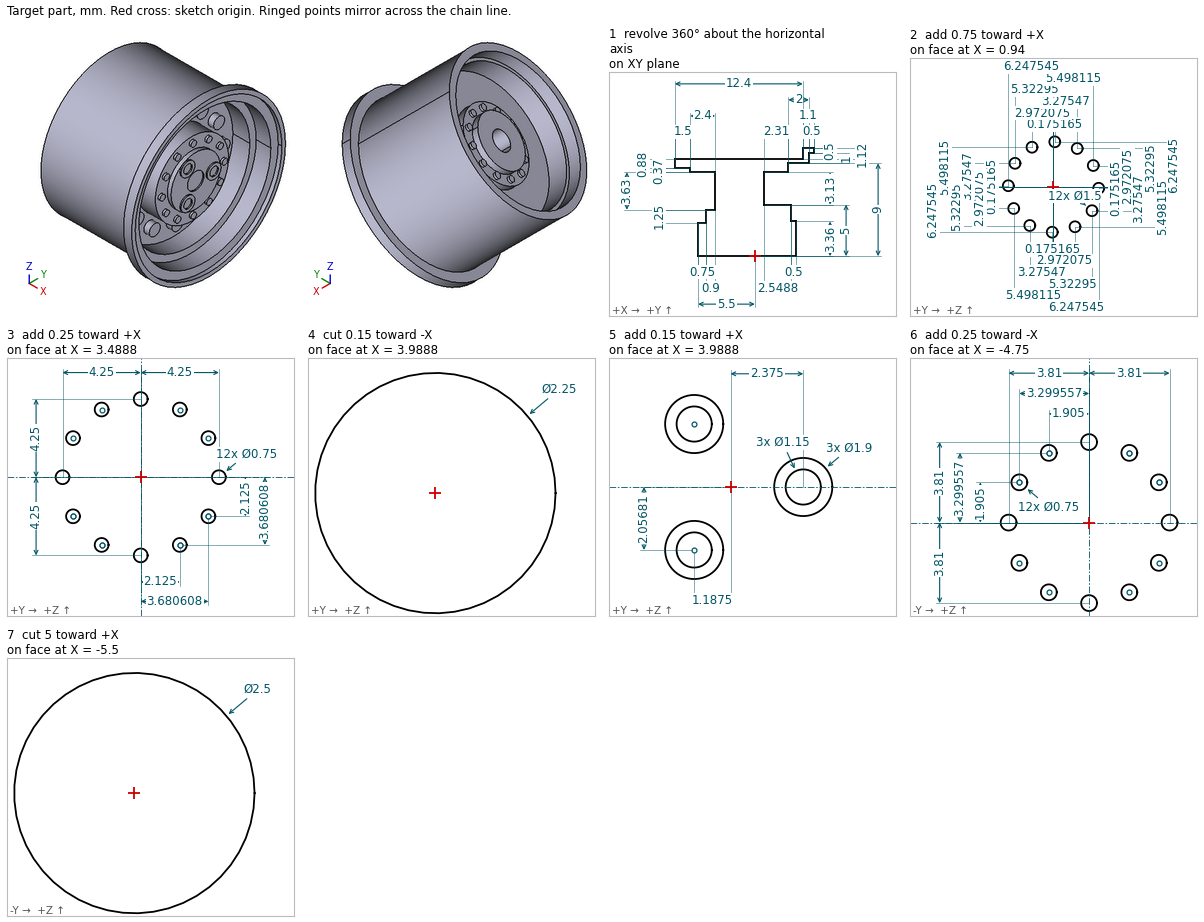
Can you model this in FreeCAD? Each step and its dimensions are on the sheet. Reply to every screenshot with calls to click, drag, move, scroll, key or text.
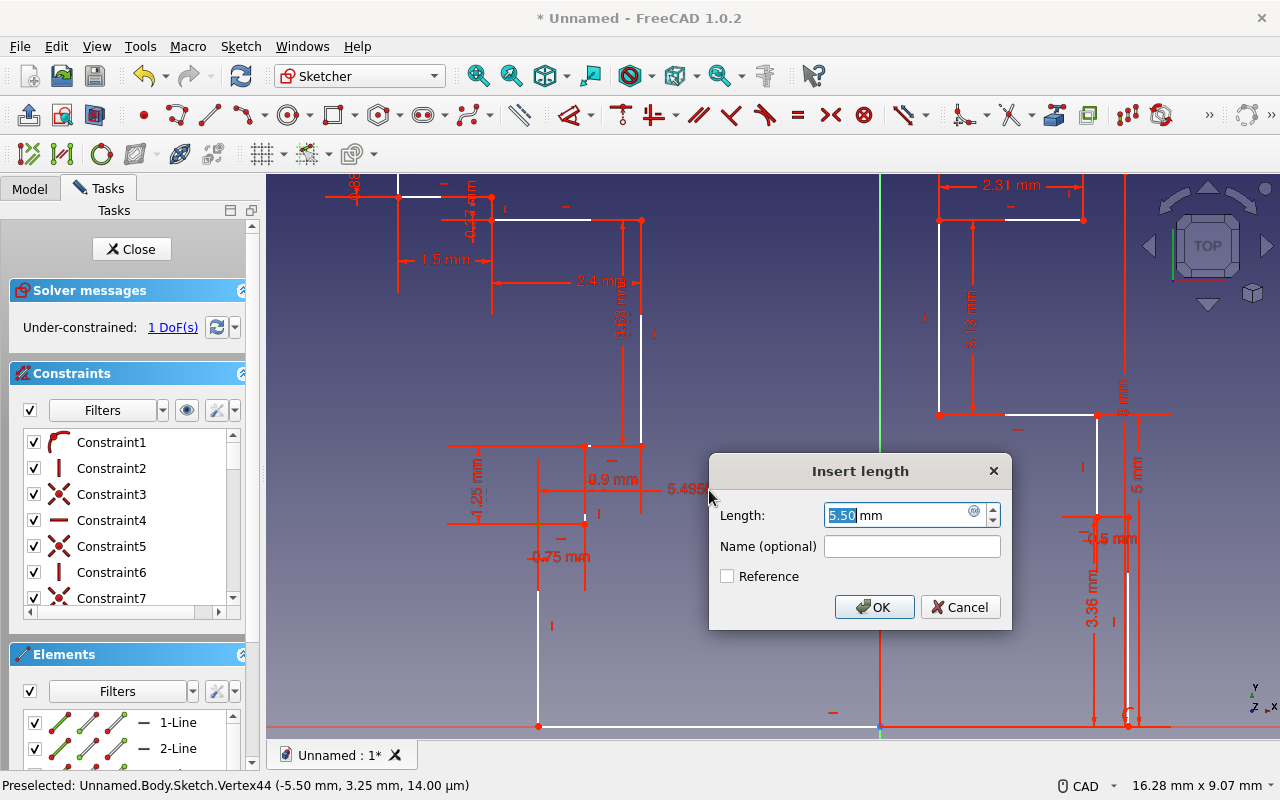
text(5.5)
key(Return)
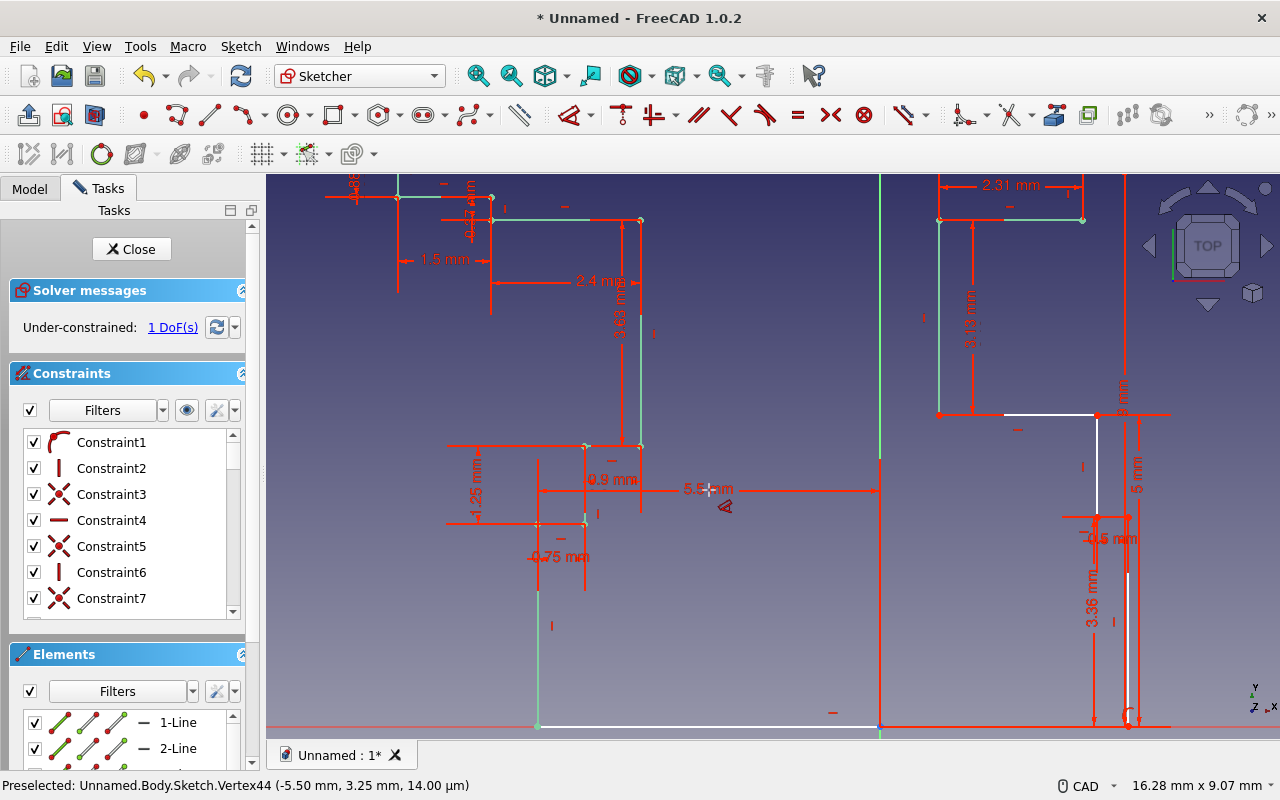
click(1050, 415)
click(1018, 449)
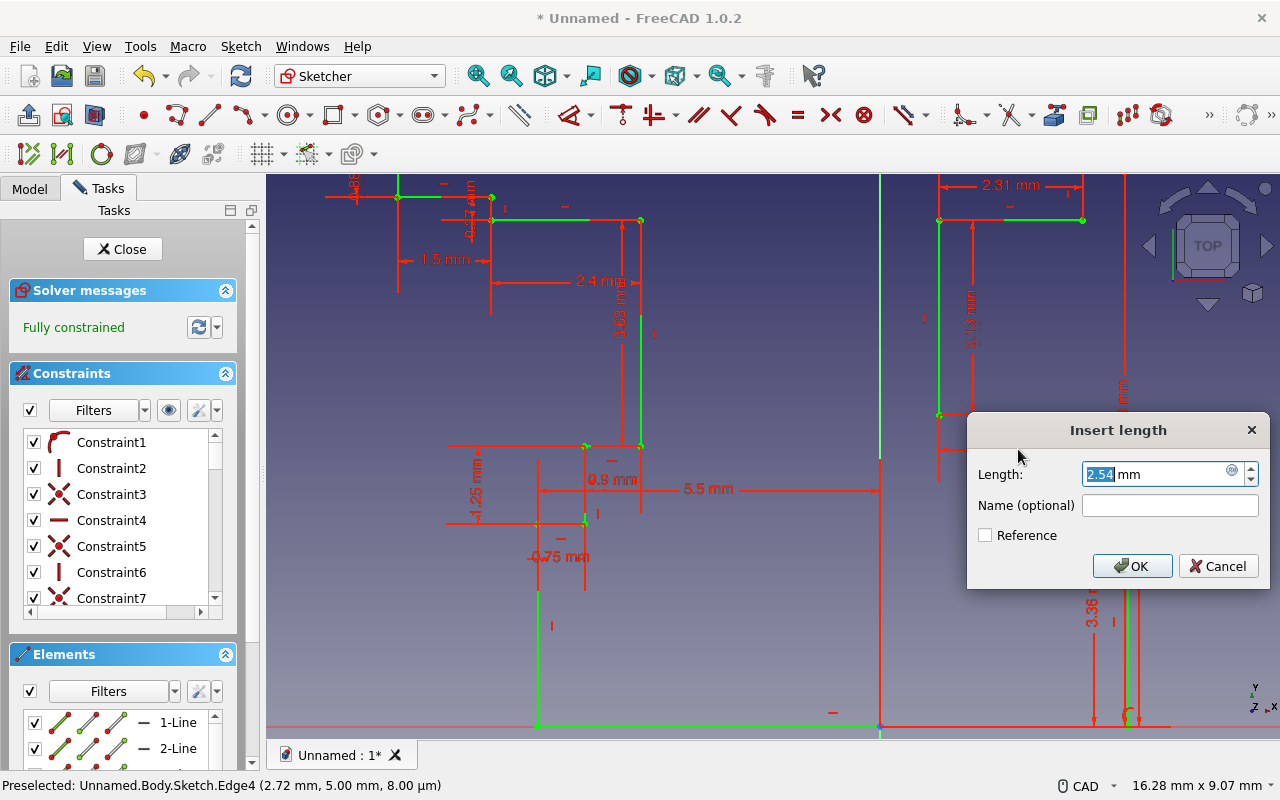
text(2.5488)
key(Return)
key(Escape)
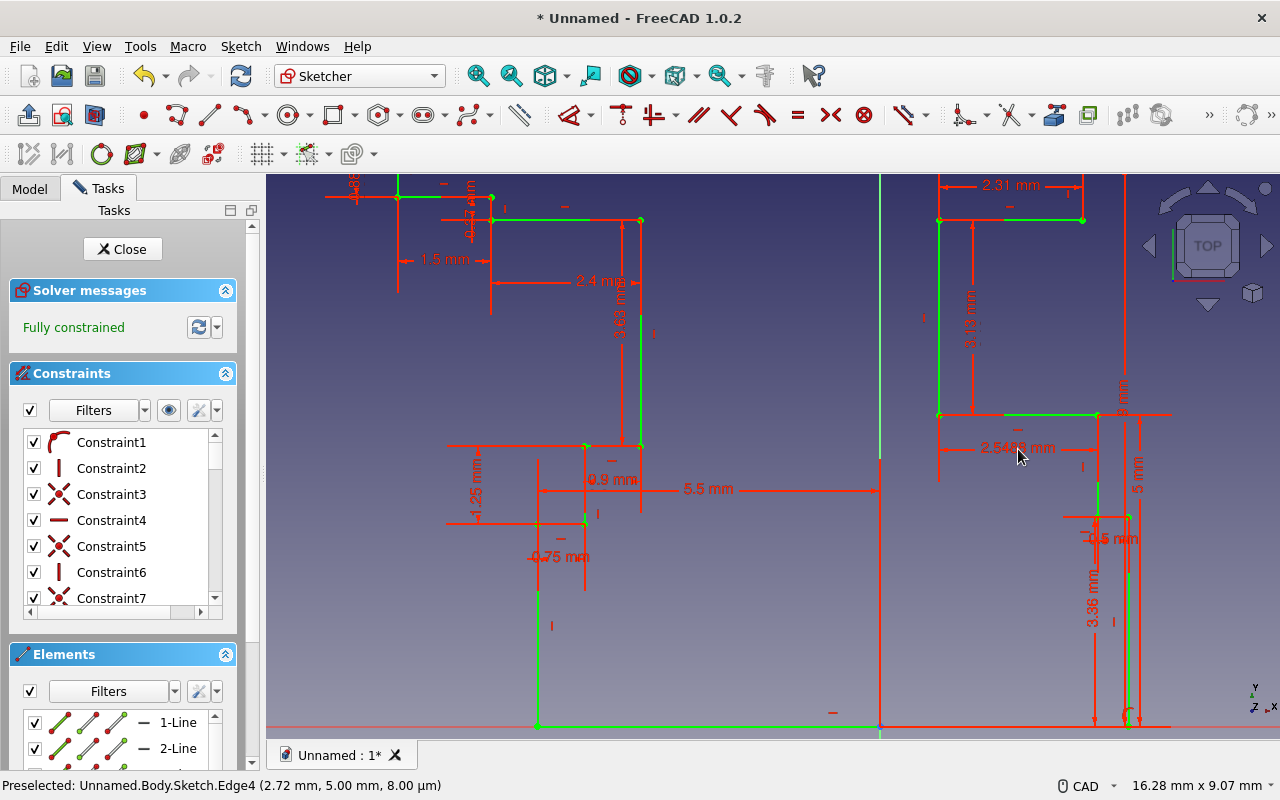
click(123, 249)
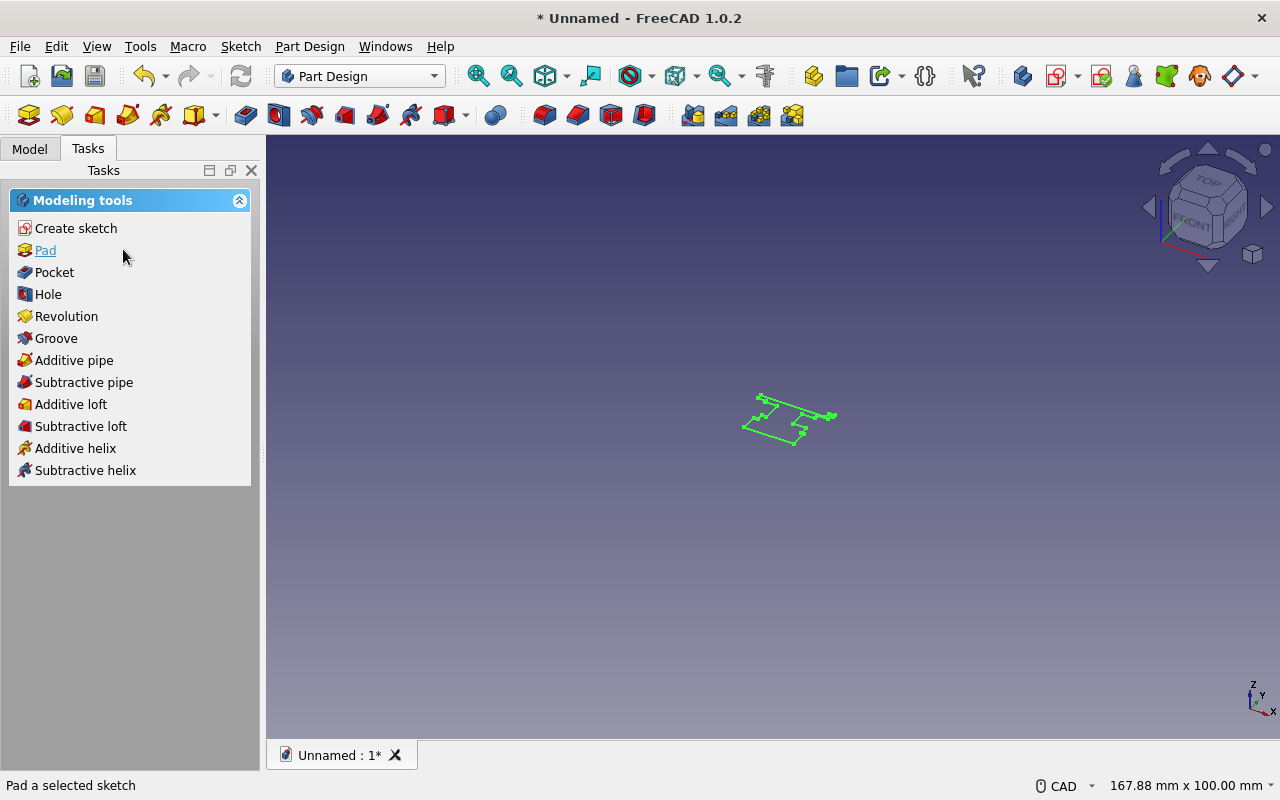
click(62, 116)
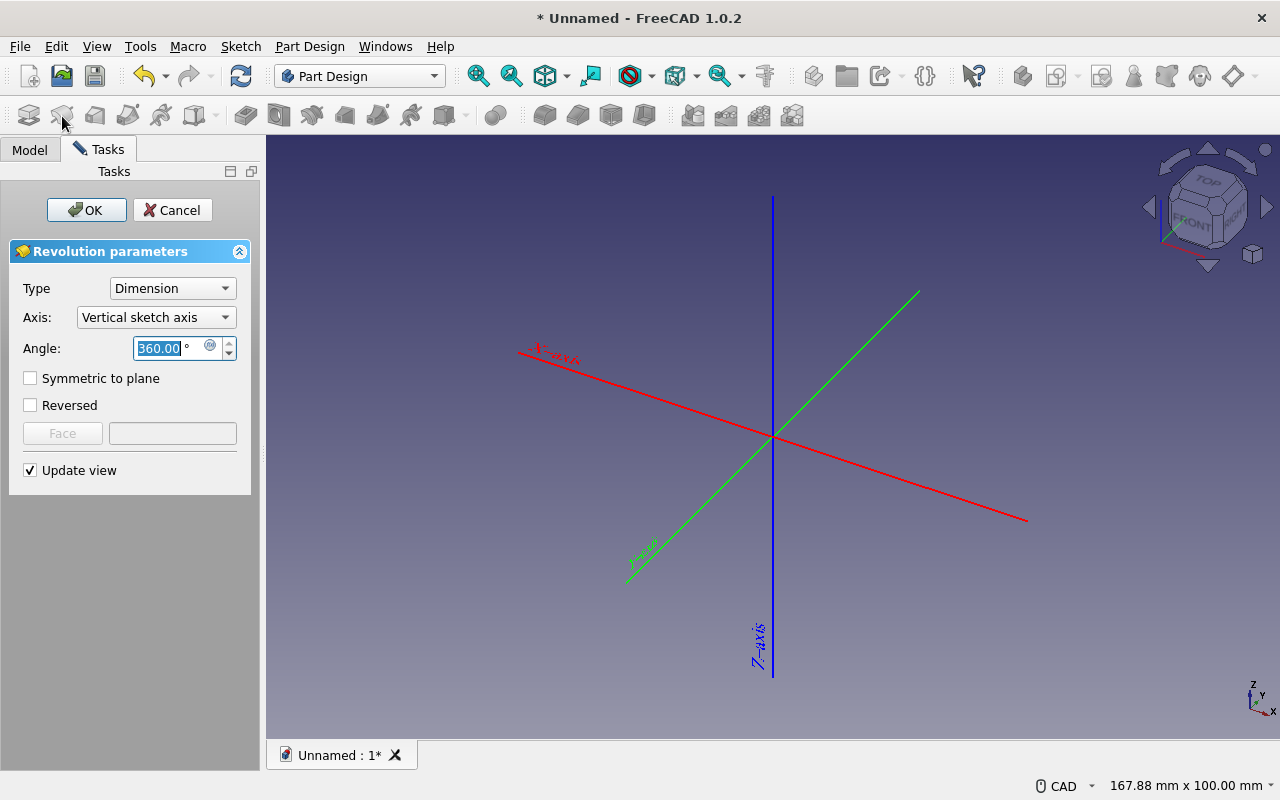
click(157, 318)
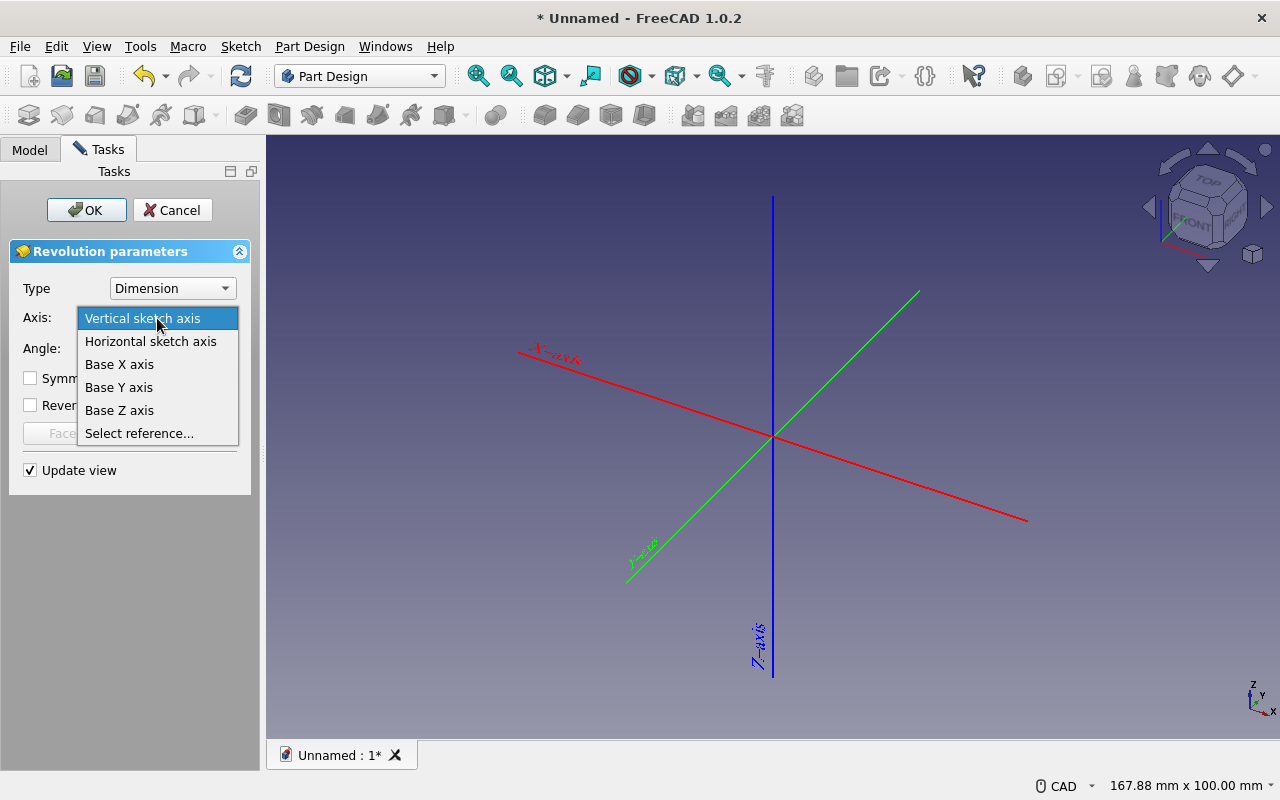
click(156, 342)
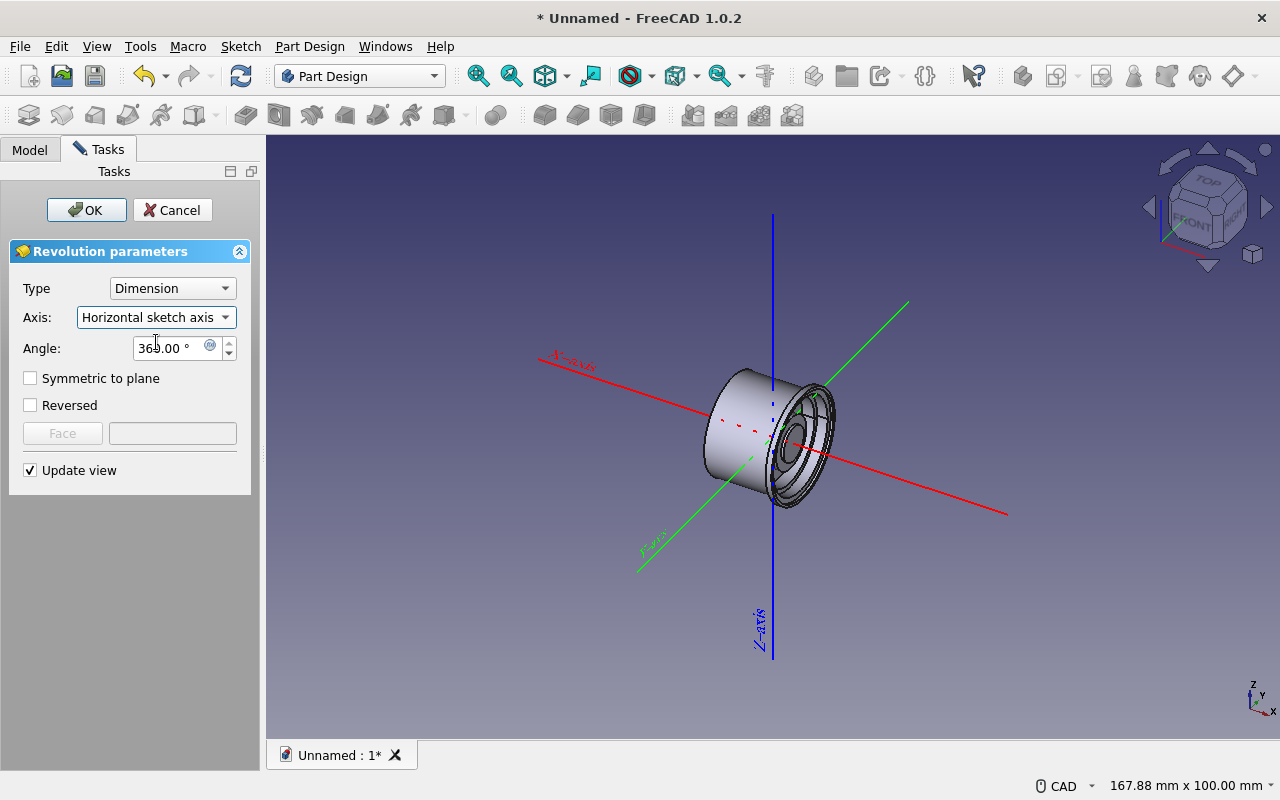
click(87, 210)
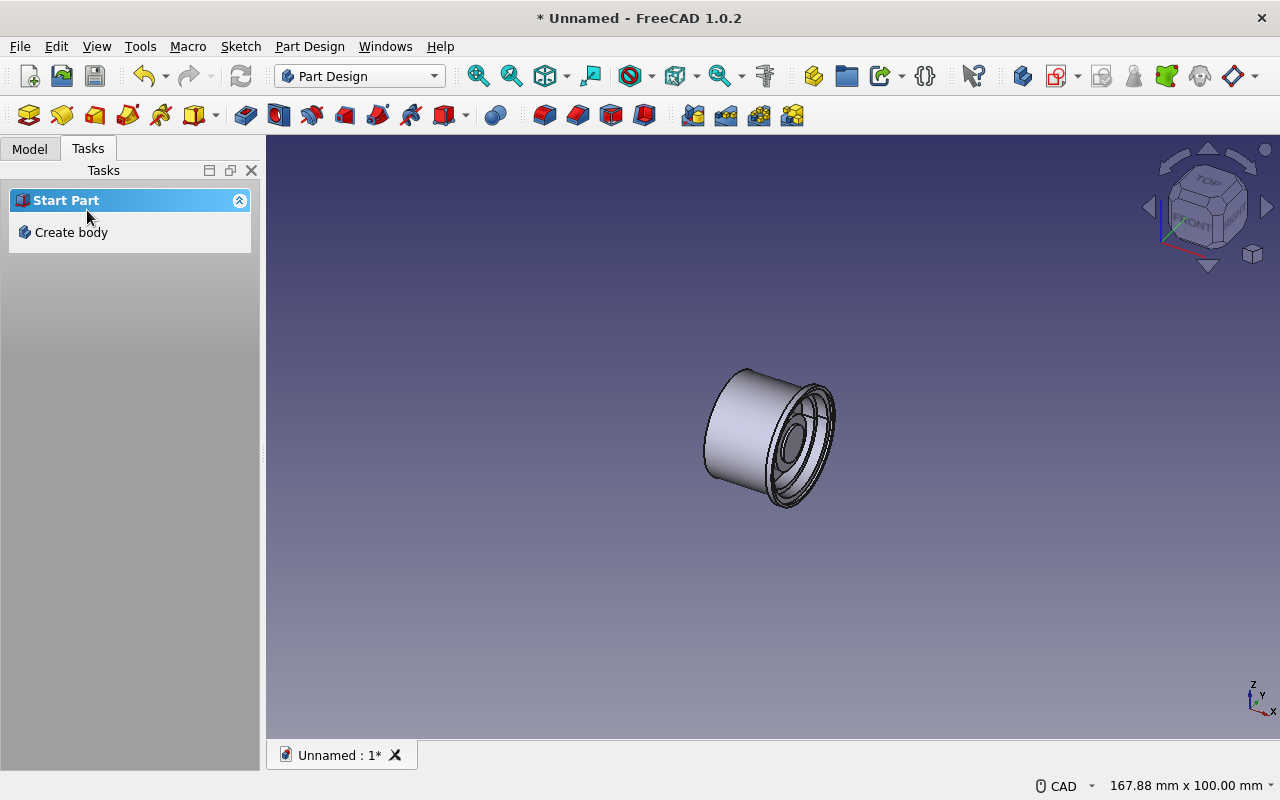
click(479, 76)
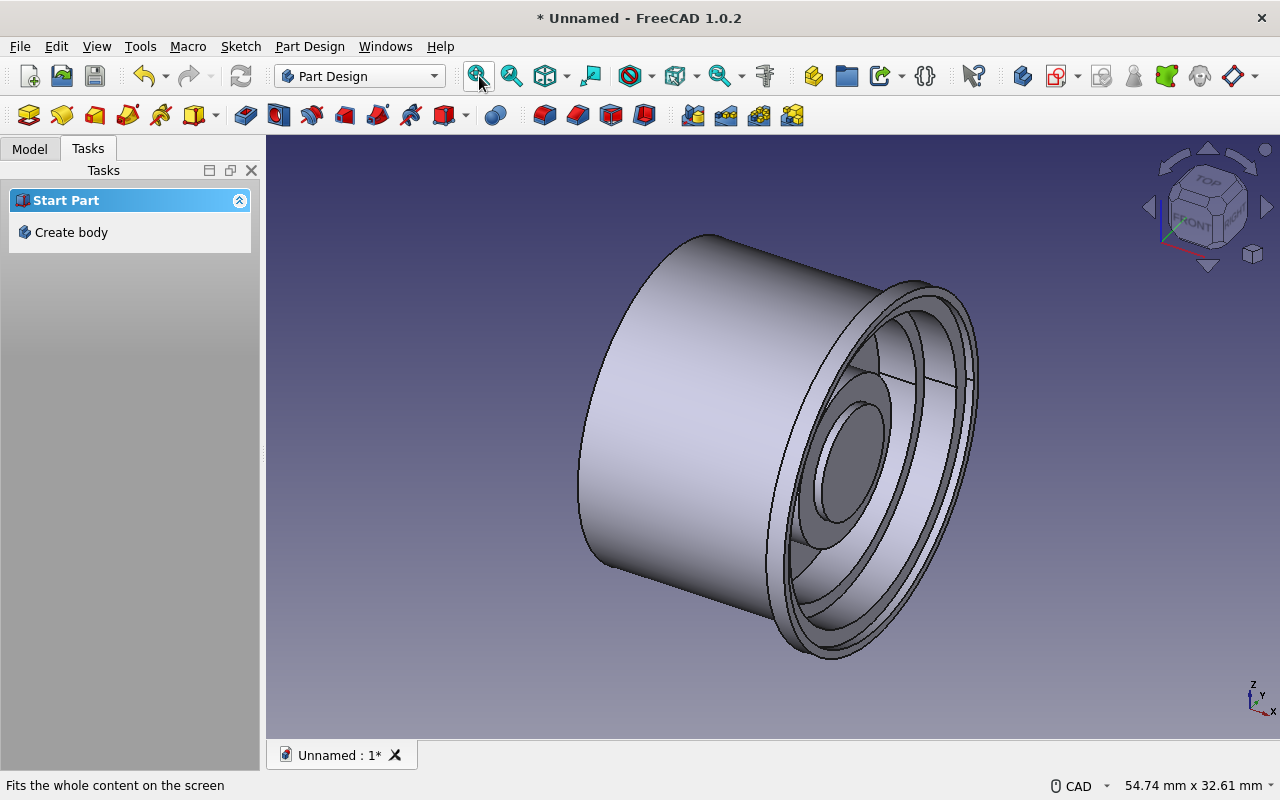
click(804, 552)